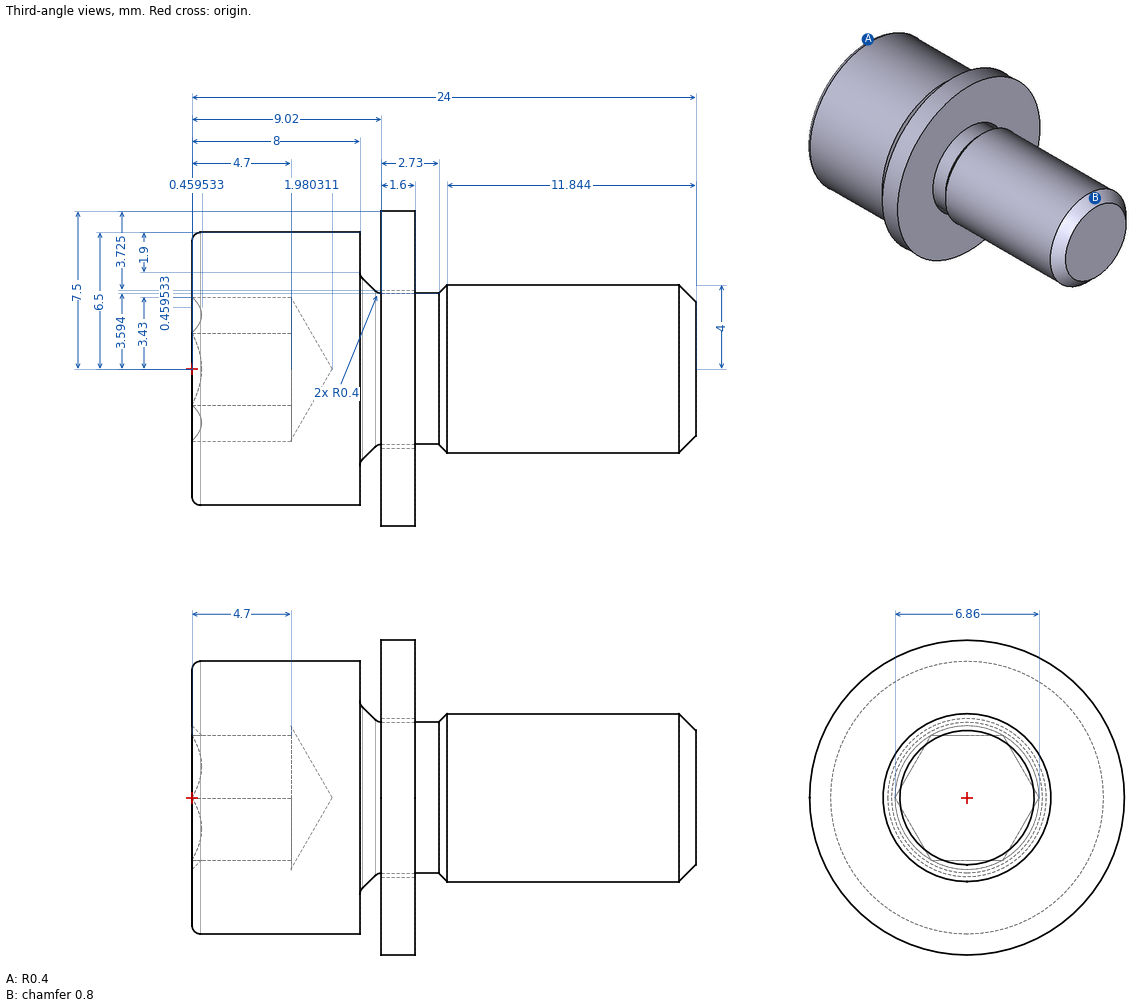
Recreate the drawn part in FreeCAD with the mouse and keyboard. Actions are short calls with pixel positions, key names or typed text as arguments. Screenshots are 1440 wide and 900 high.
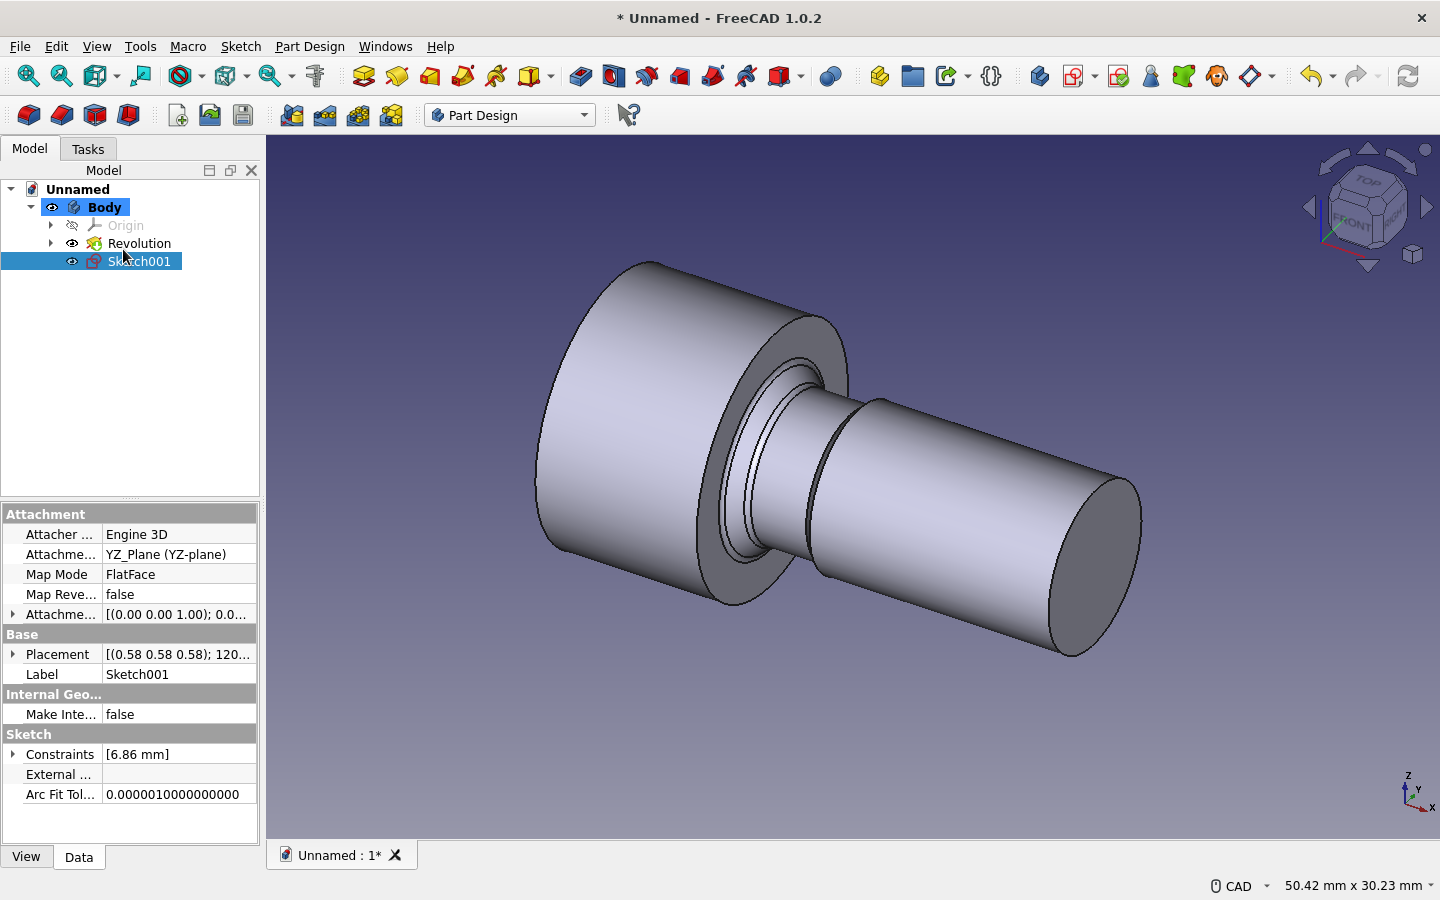
click(581, 76)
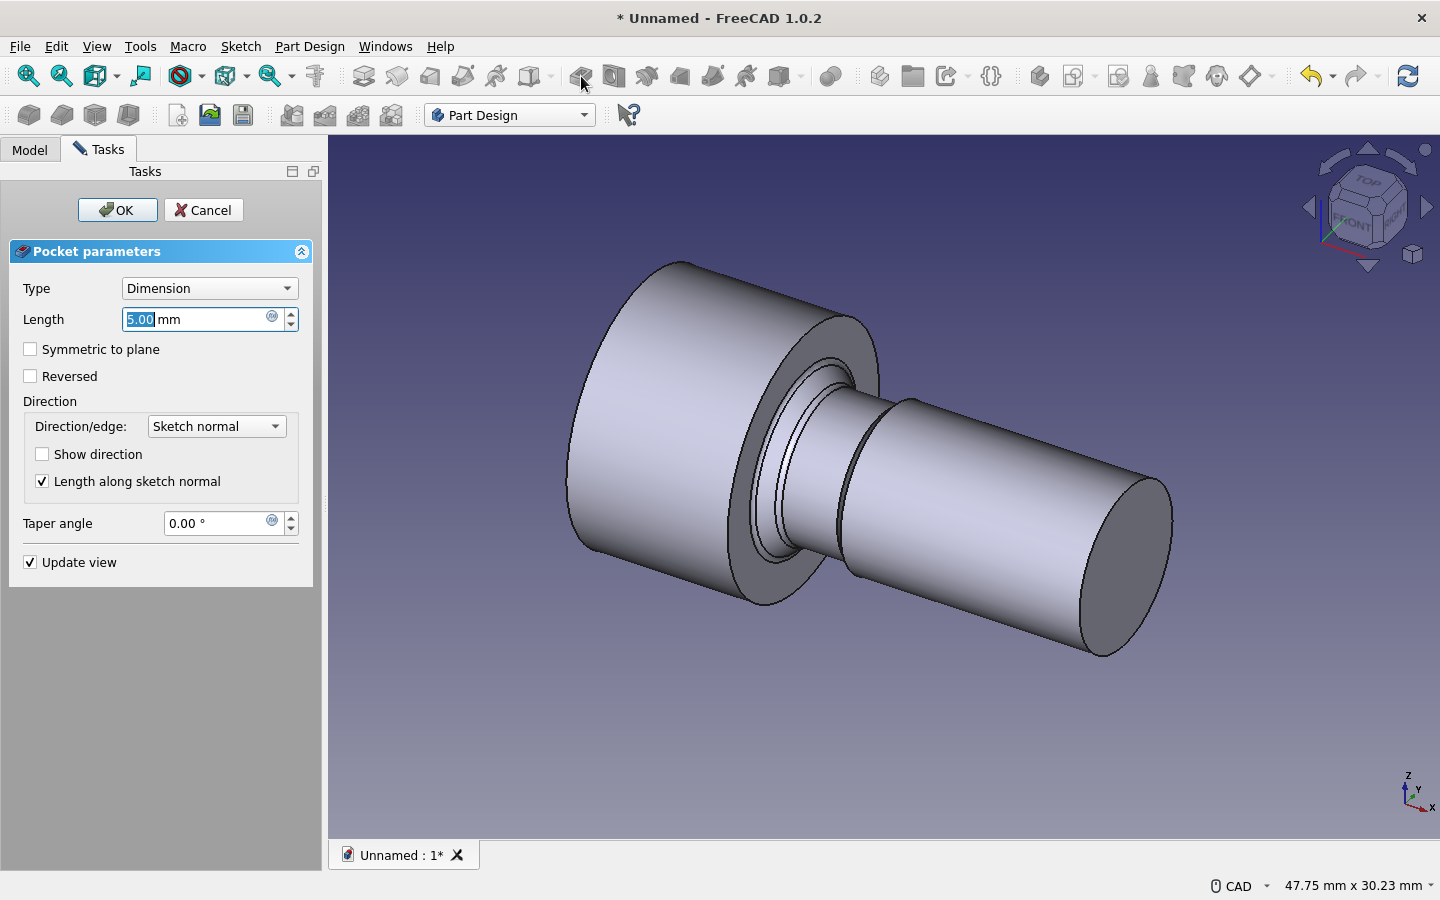
text(4.7)
key(Tab)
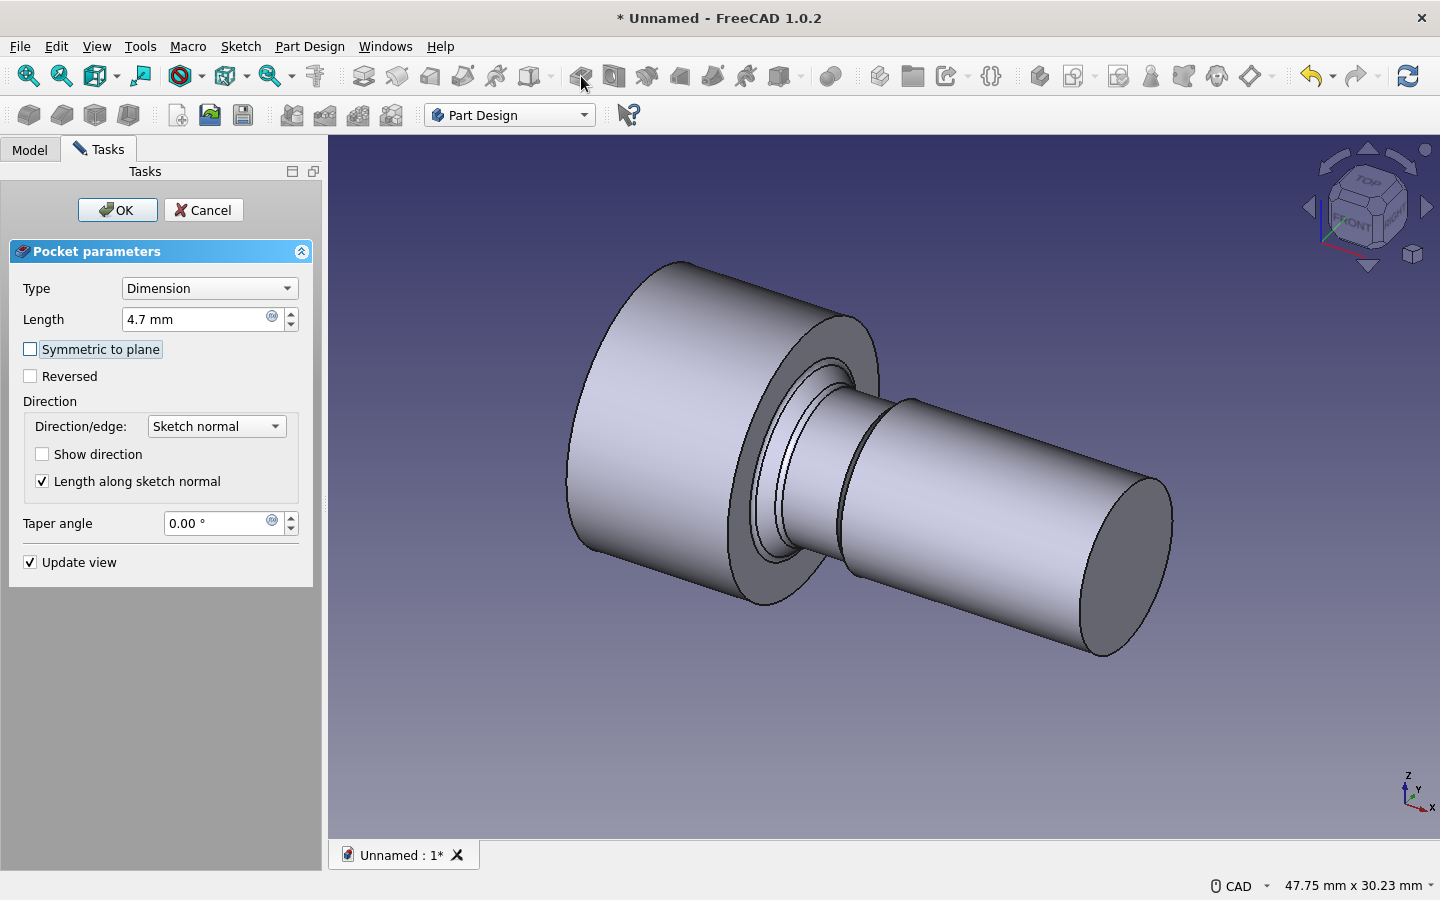
click(31, 376)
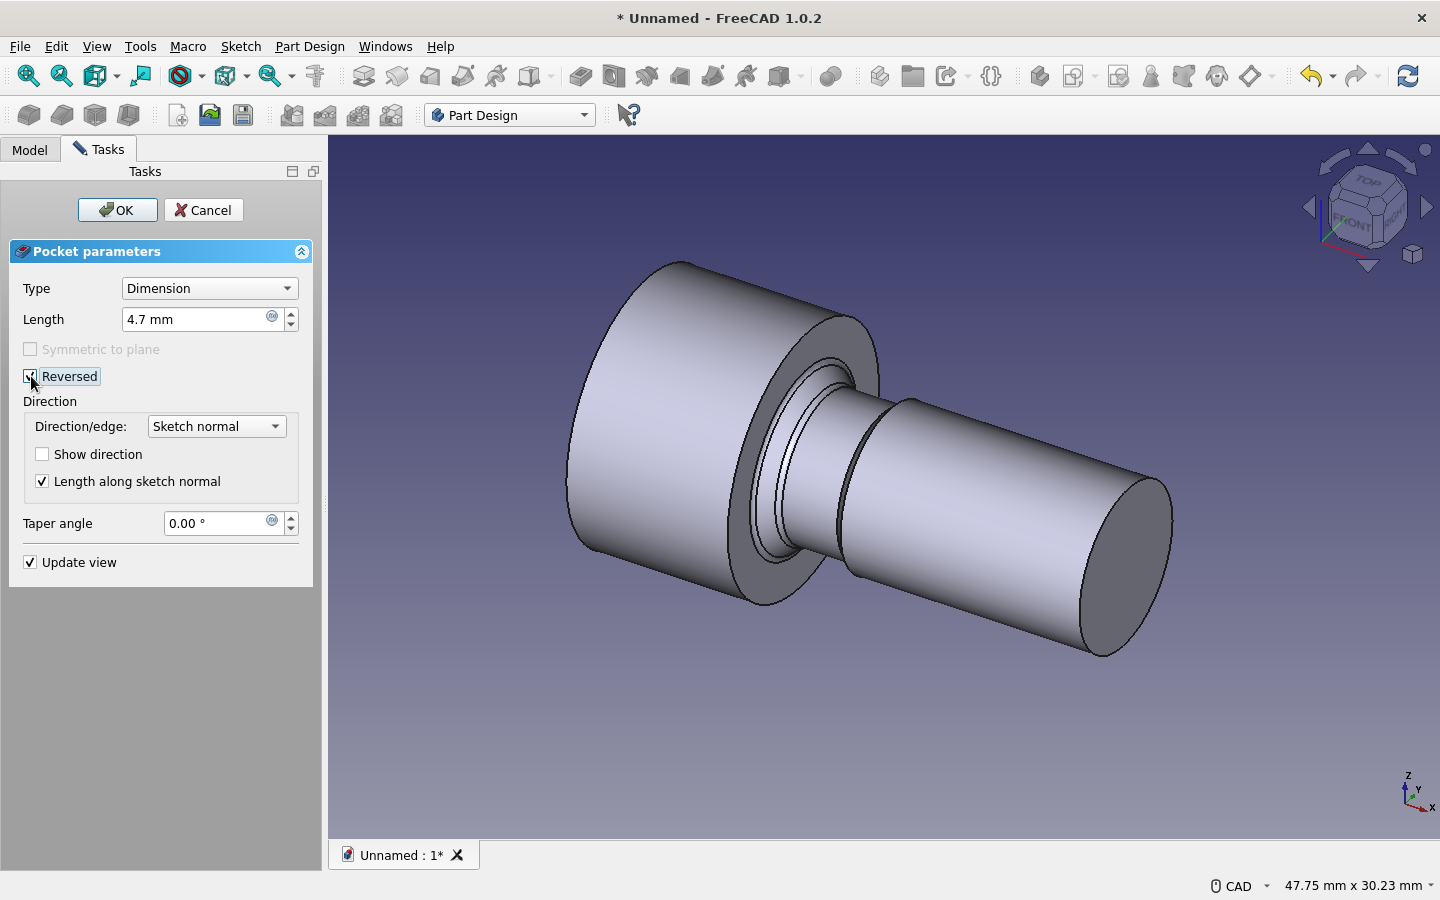
click(118, 210)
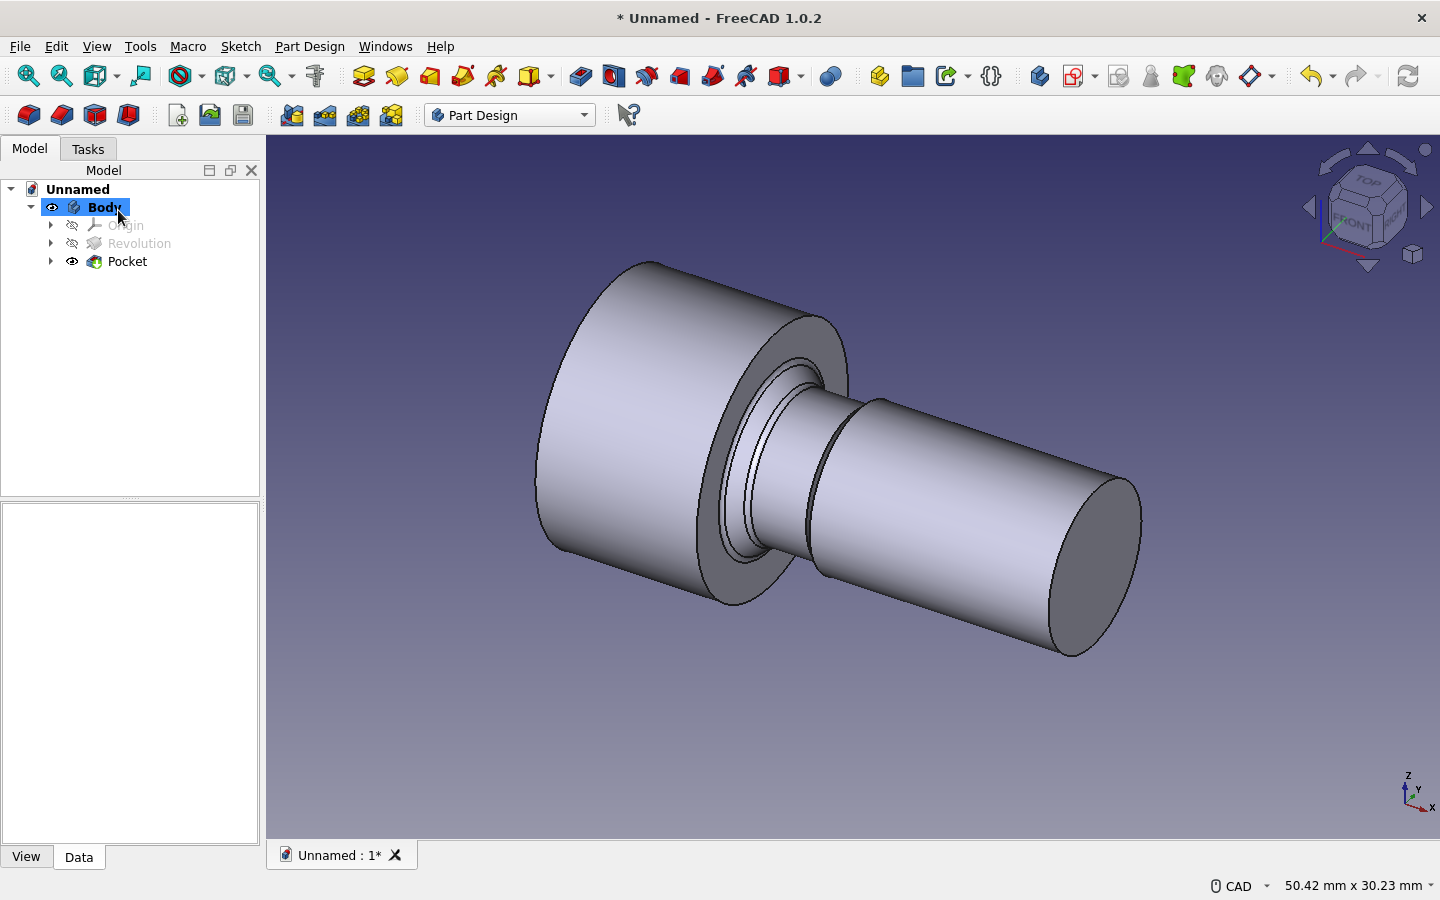
click(1072, 76)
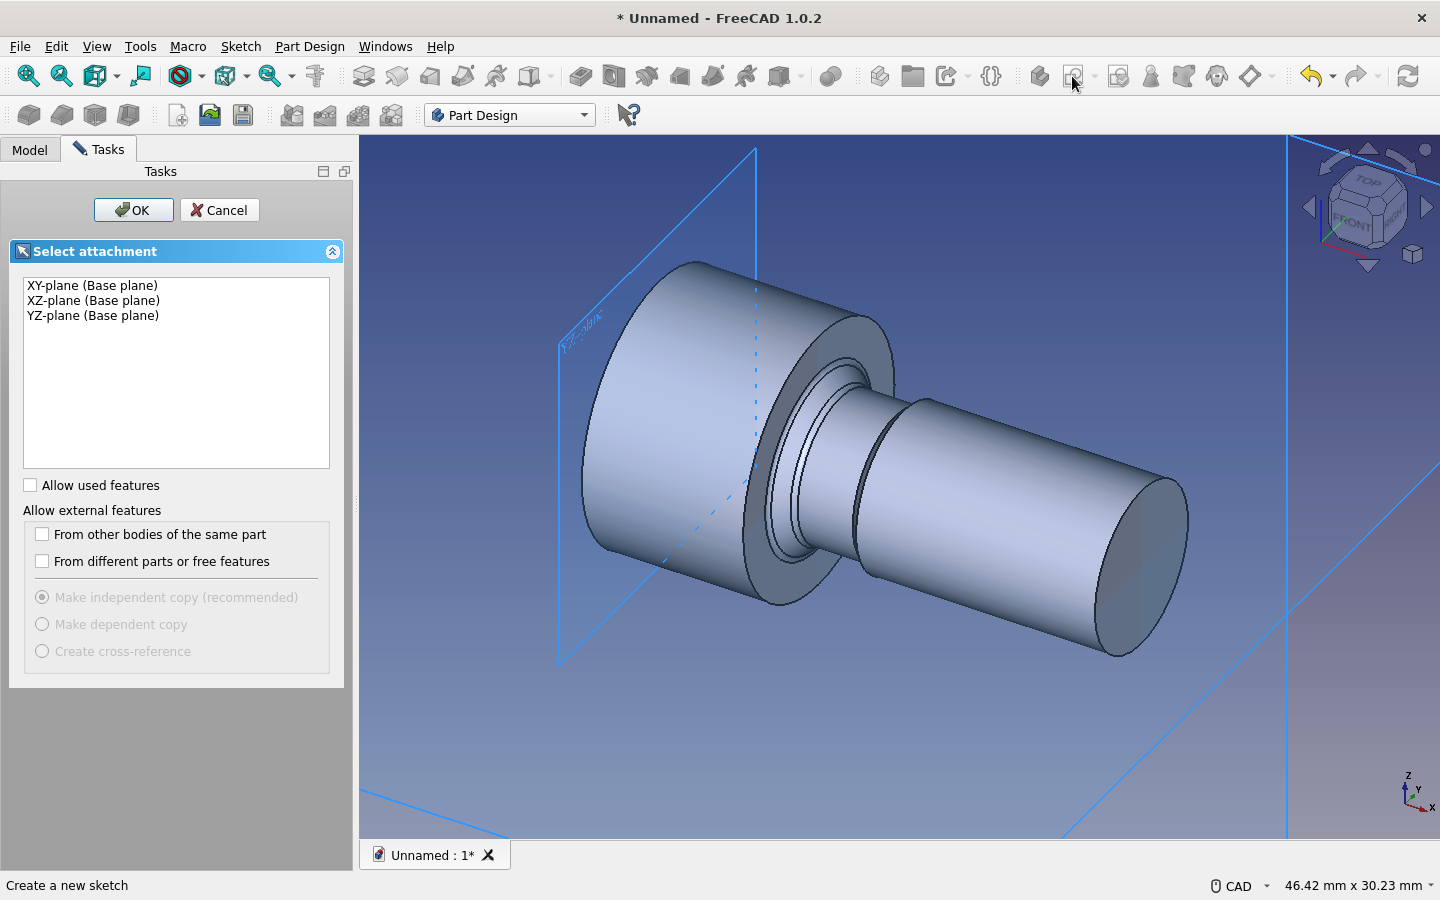
click(84, 286)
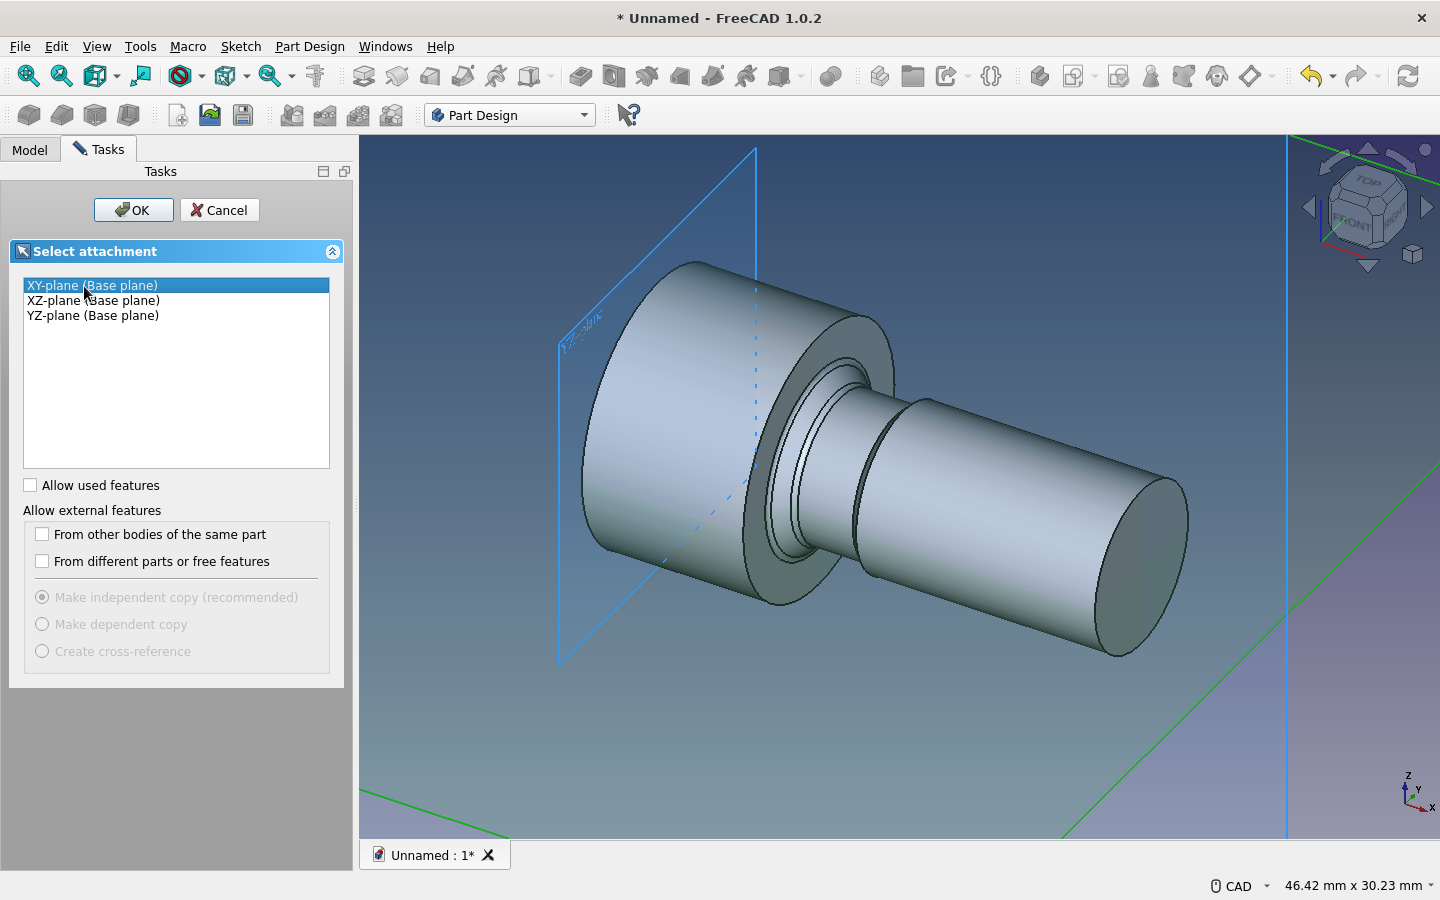
click(134, 210)